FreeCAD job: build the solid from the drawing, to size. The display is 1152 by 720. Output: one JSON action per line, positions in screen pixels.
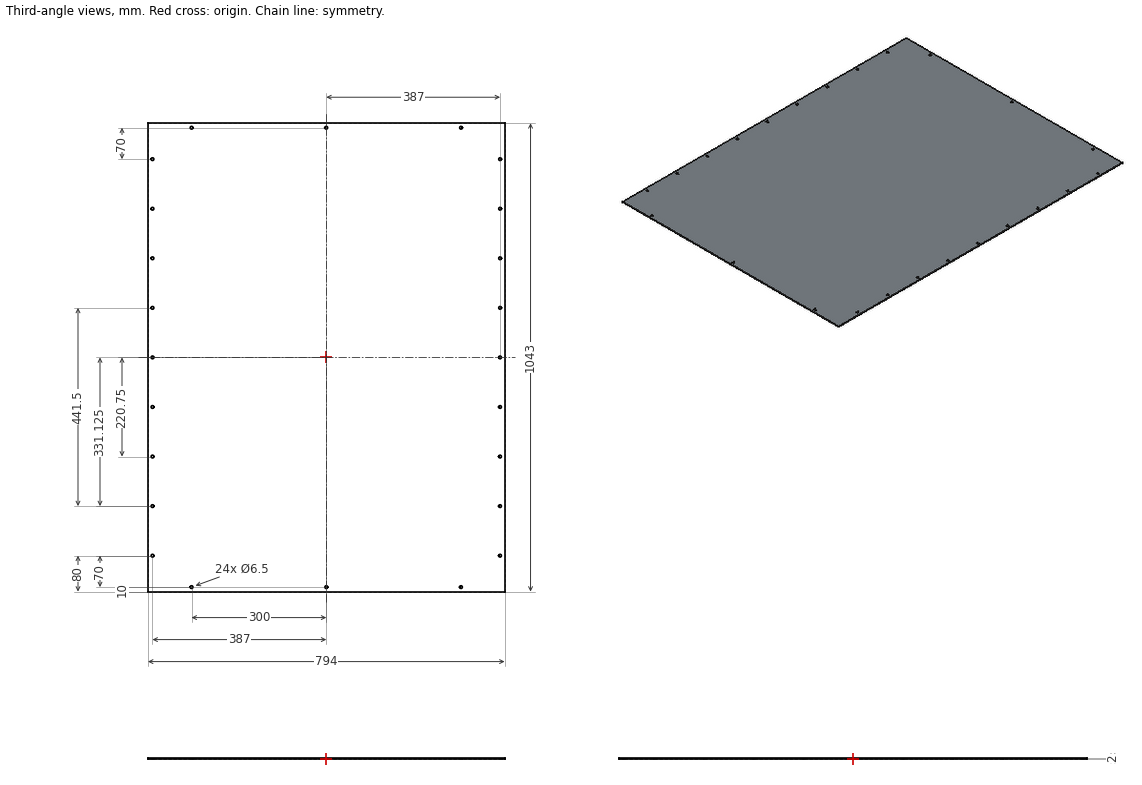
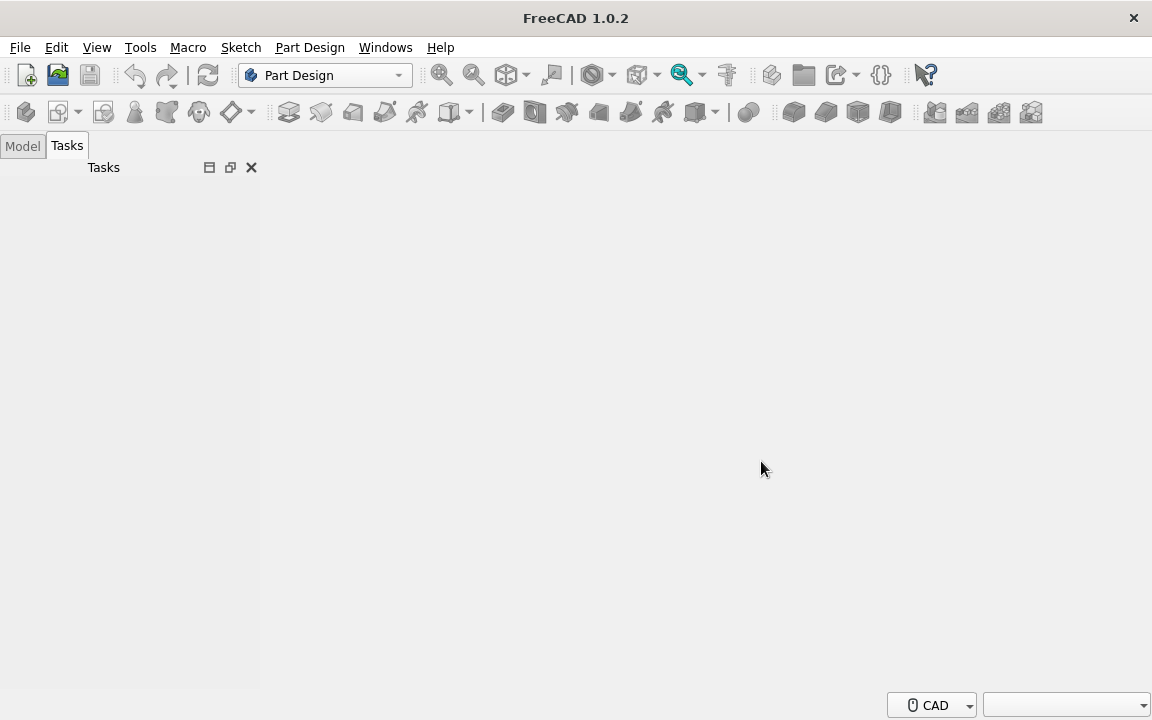
{"action": "left_click", "coordinate": [26, 76]}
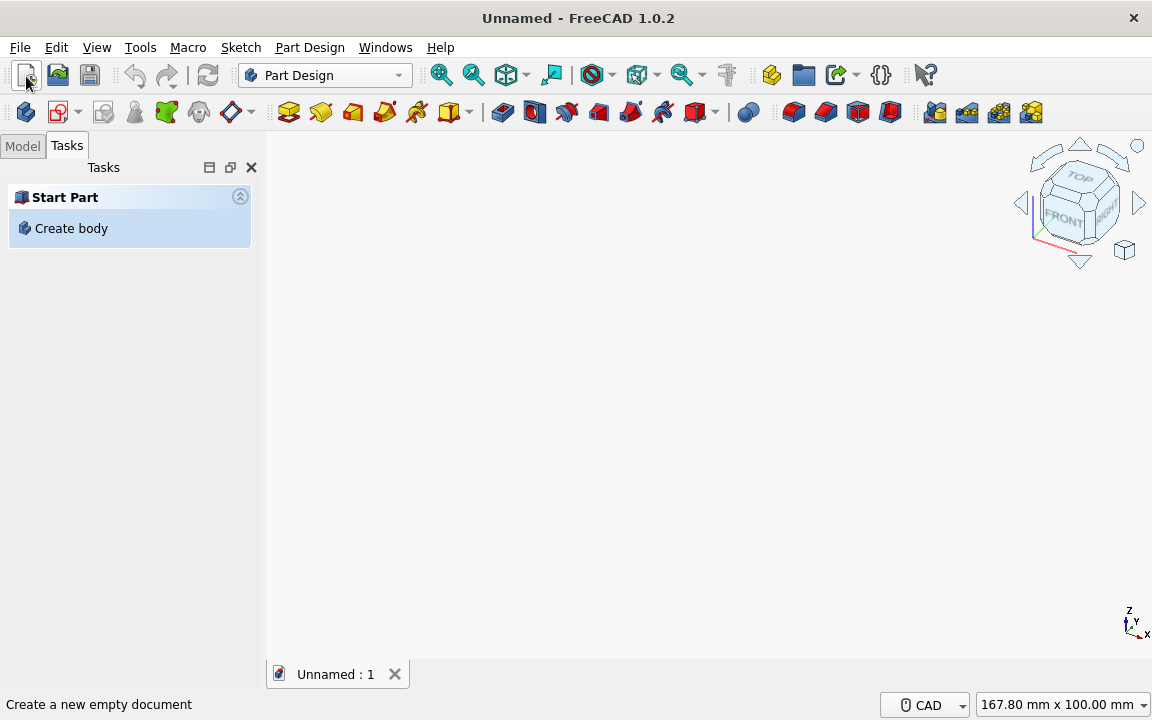
{"action": "left_click", "coordinate": [58, 112]}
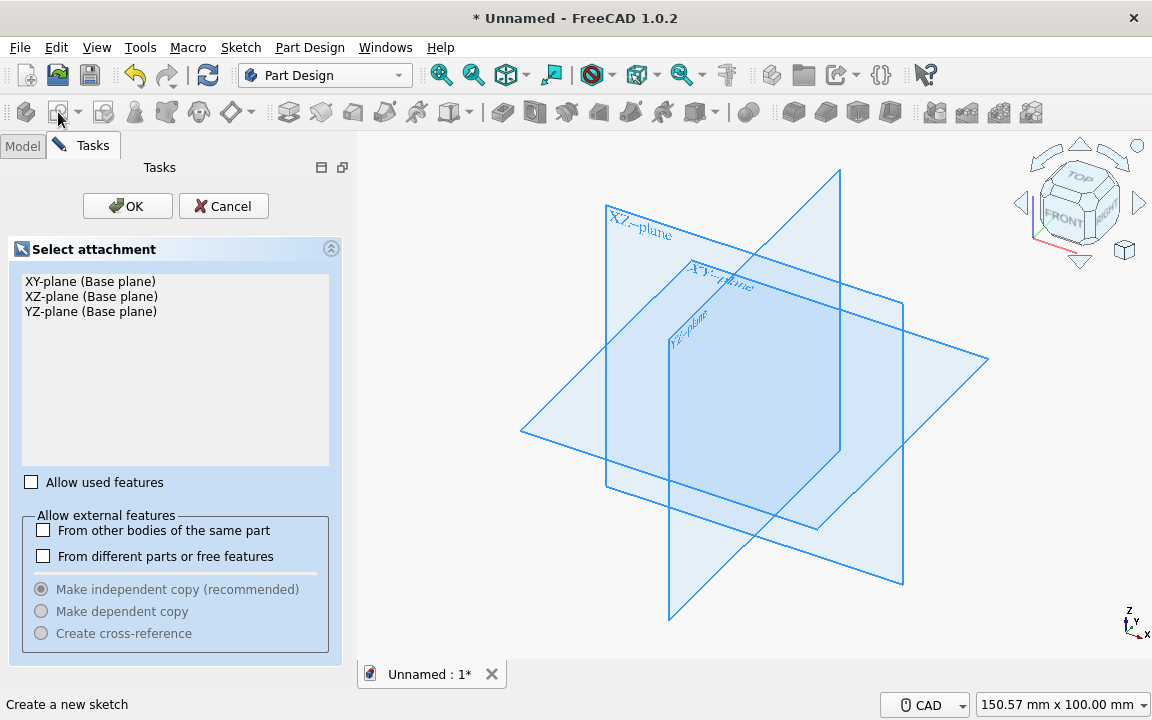
{"action": "left_click", "coordinate": [82, 282]}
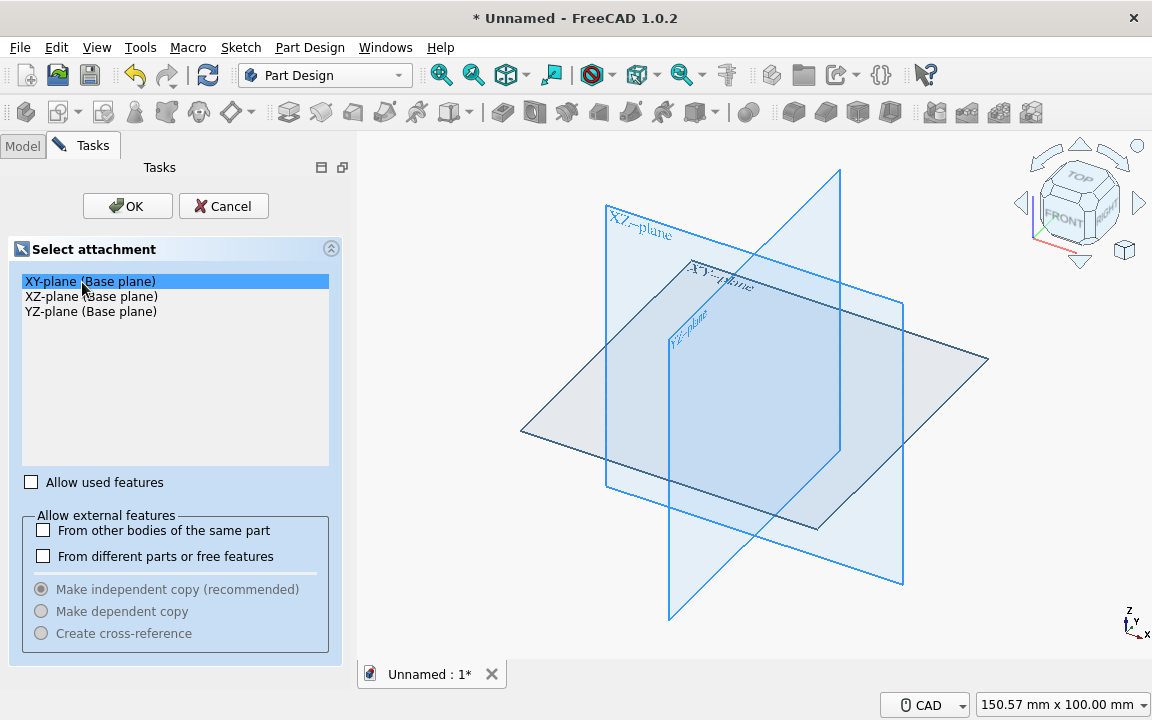
{"action": "left_click", "coordinate": [128, 206]}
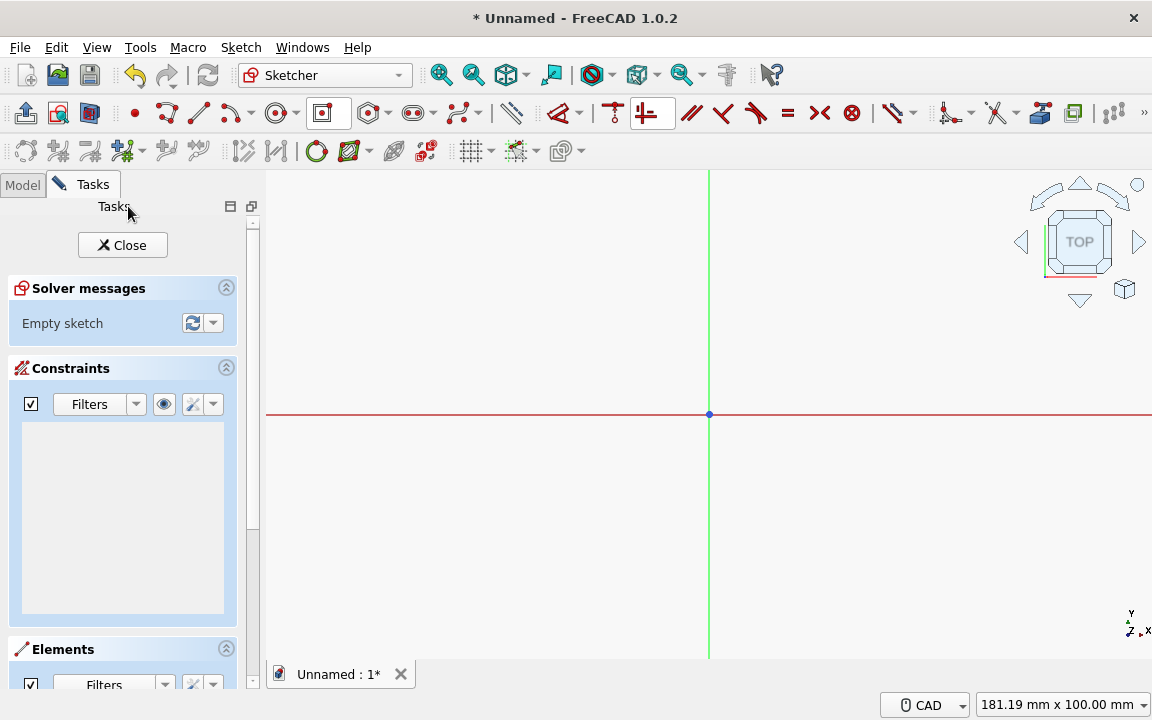
{"action": "scroll", "coordinate": [636, 414], "scroll_direction": "down", "scroll_amount": 14}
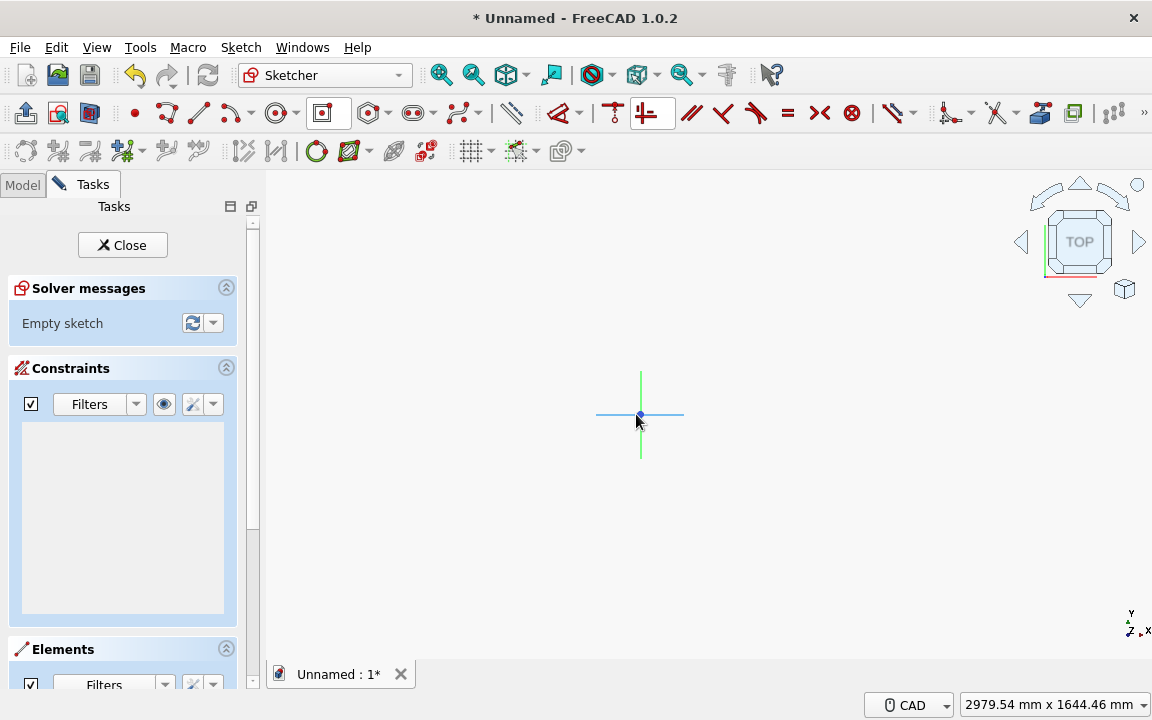
{"action": "left_click", "coordinate": [322, 114]}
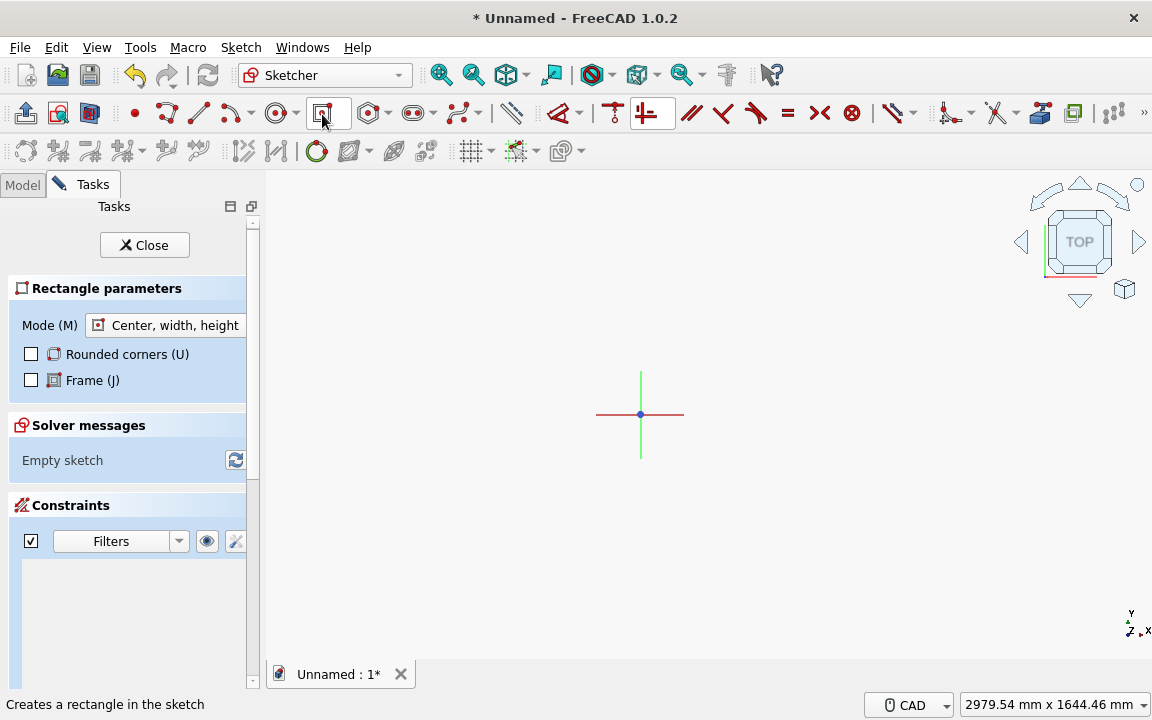
{"action": "left_click", "coordinate": [641, 414]}
{"action": "mouse_move", "coordinate": [759, 259]}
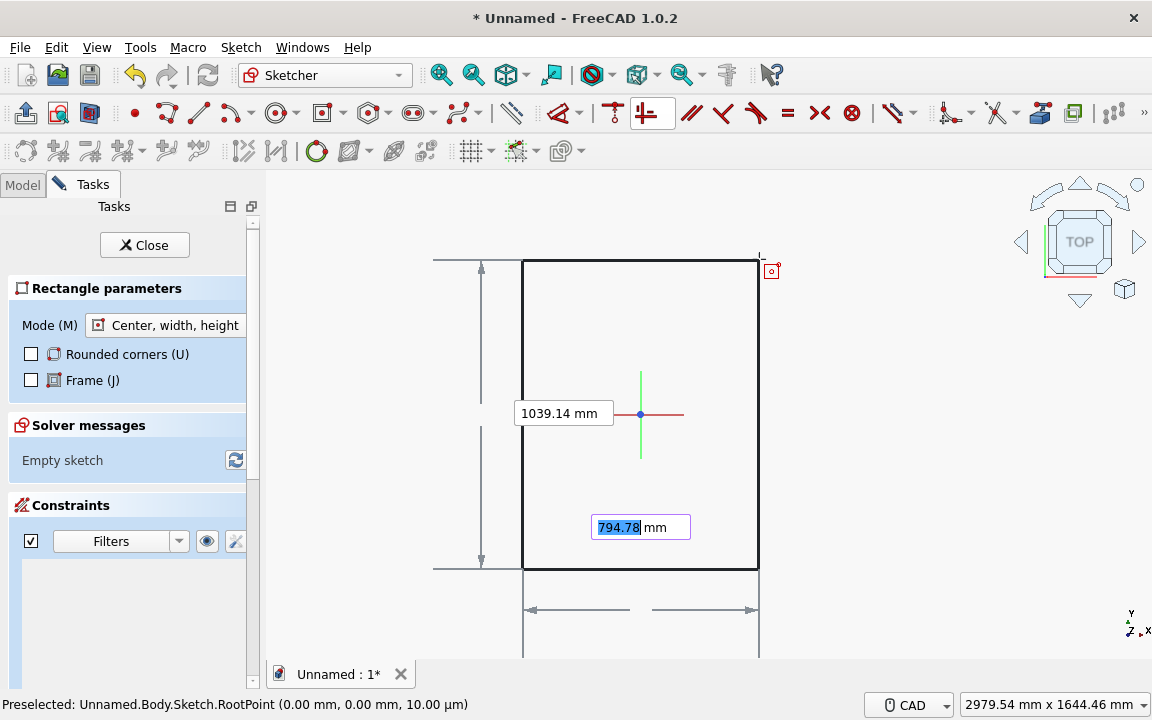
{"action": "type", "text": "794"}
{"action": "key", "text": "Tab"}
{"action": "type", "text": "1043"}
{"action": "key", "text": "Return"}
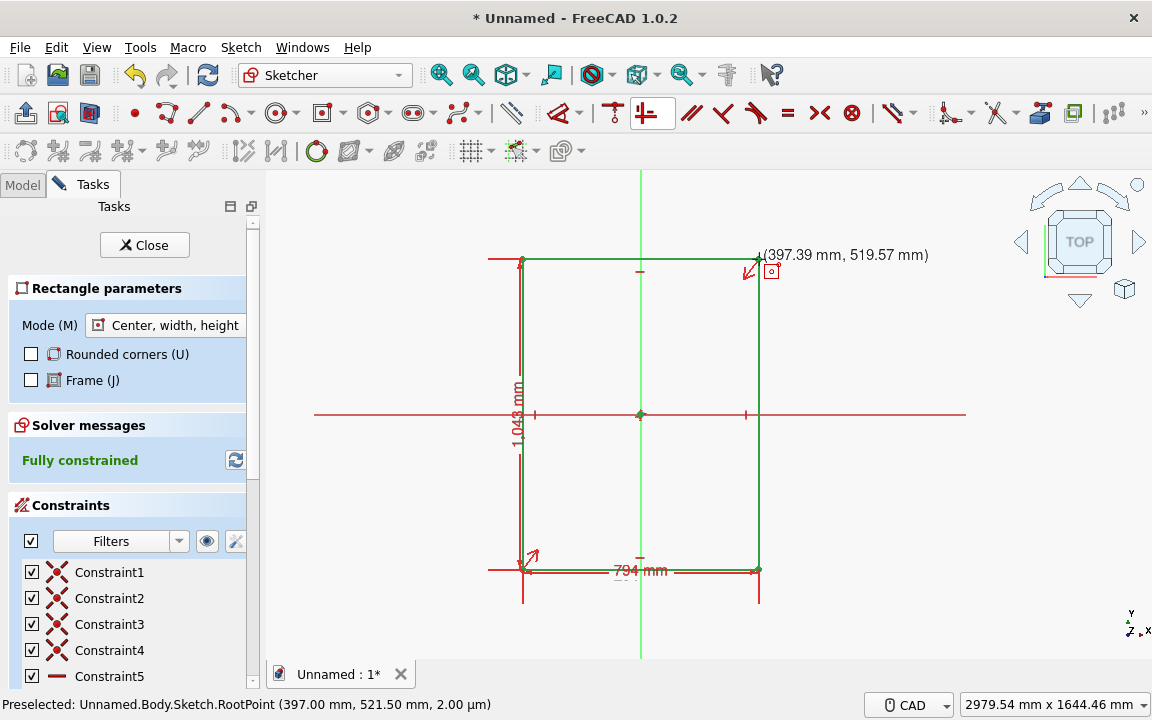
{"action": "left_click", "coordinate": [276, 114]}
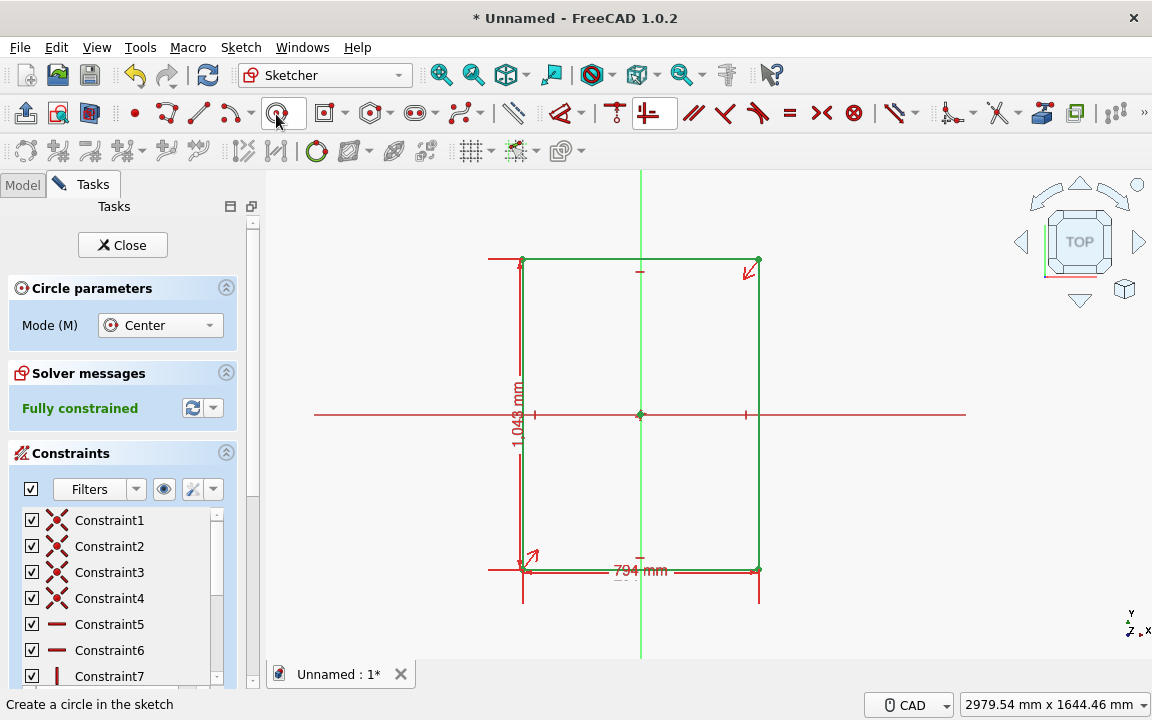
{"action": "scroll", "coordinate": [552, 567], "scroll_direction": "up", "scroll_amount": 16}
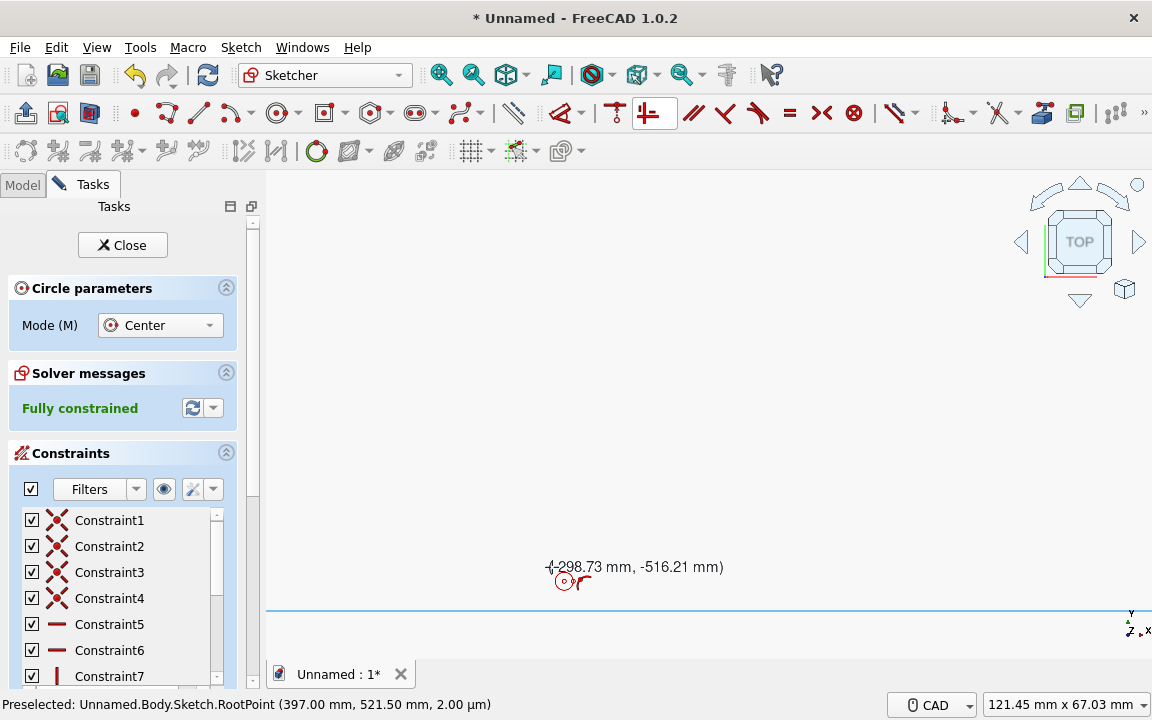
{"action": "scroll", "coordinate": [531, 604], "scroll_direction": "down", "scroll_amount": 15}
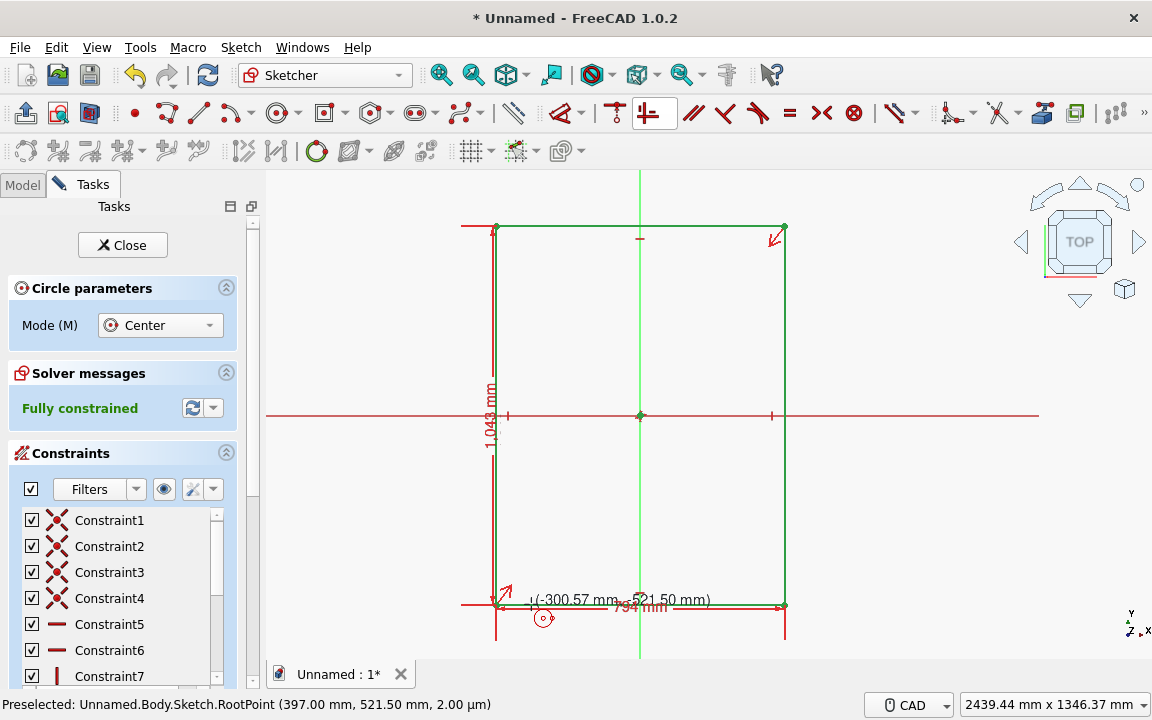
{"action": "scroll", "coordinate": [531, 602], "scroll_direction": "up", "scroll_amount": 8}